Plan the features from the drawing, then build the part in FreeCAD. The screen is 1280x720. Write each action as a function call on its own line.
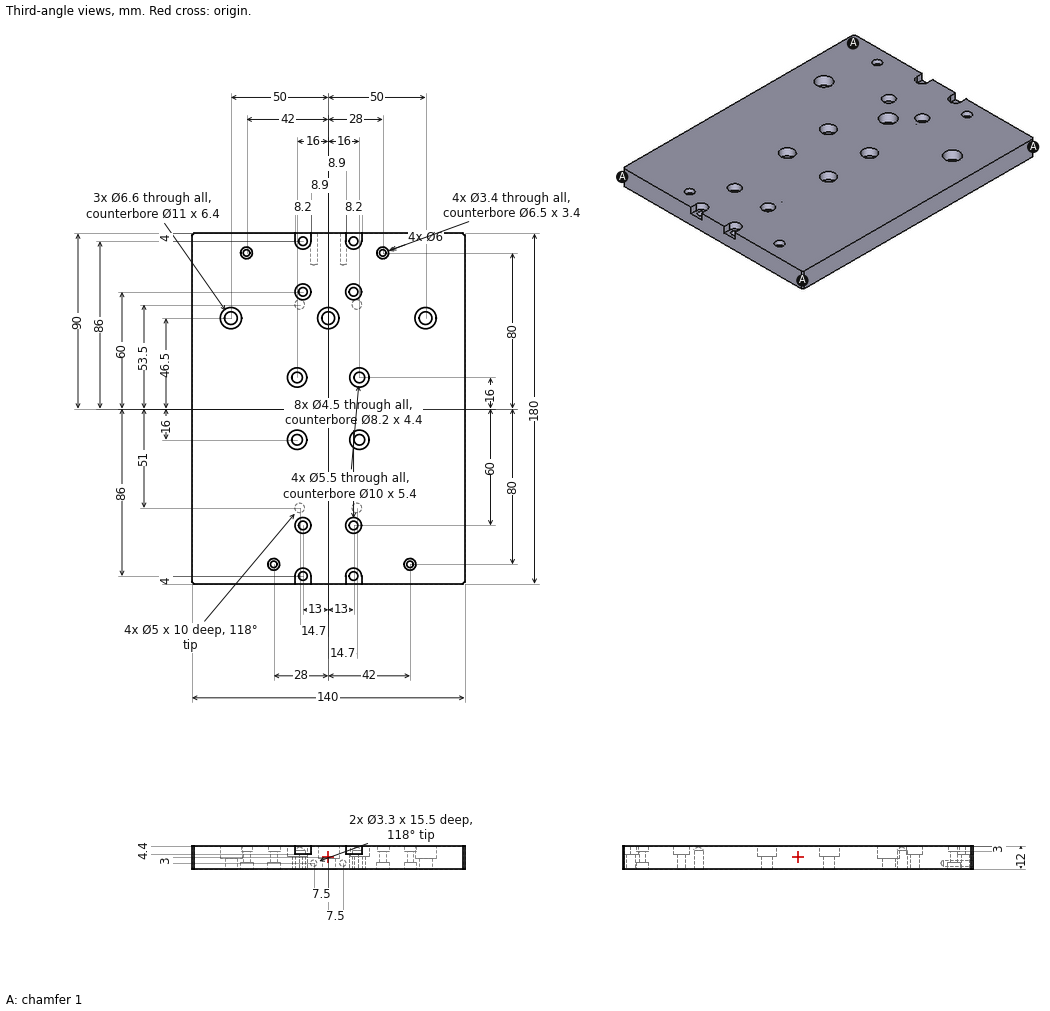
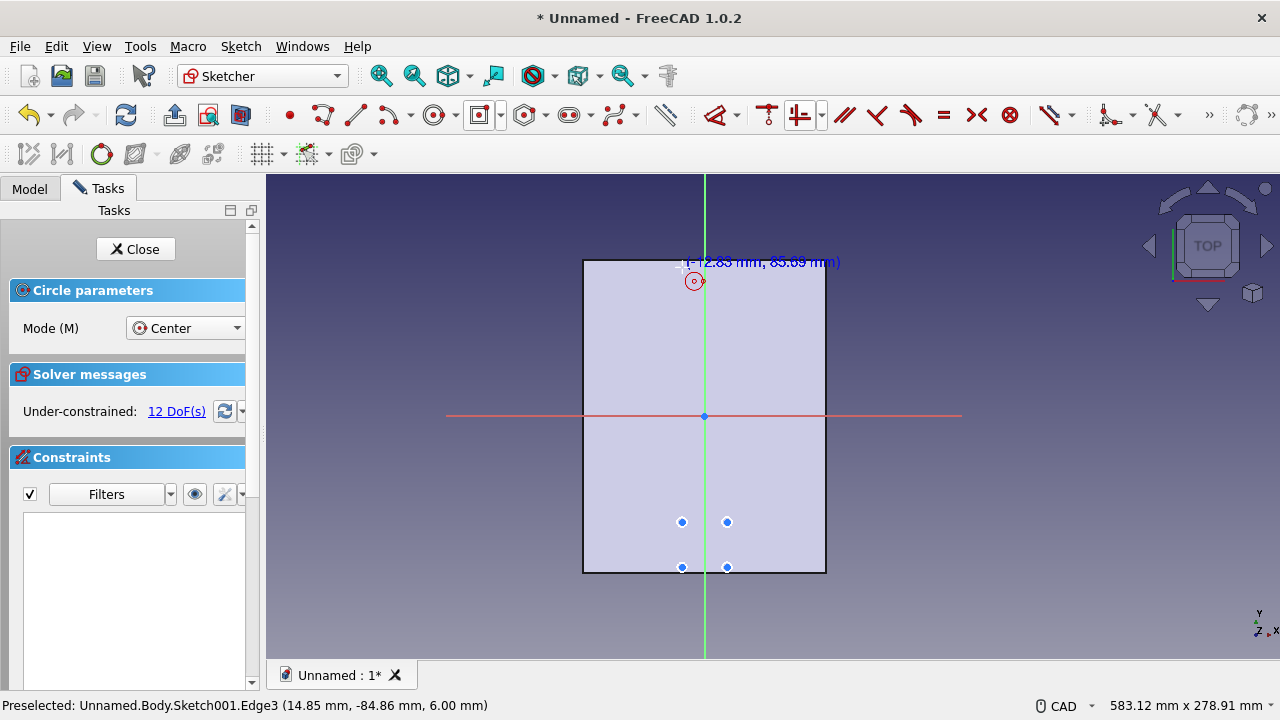
click(682, 267)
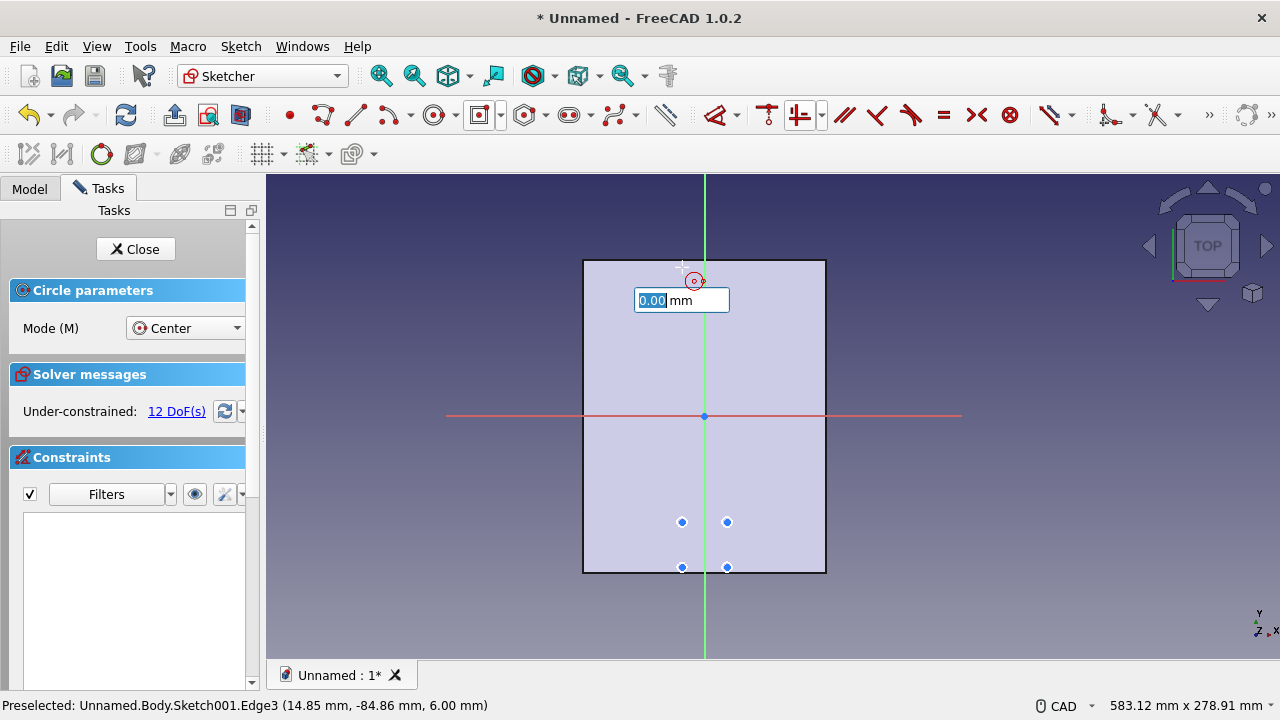
scroll(685, 264, up, 8)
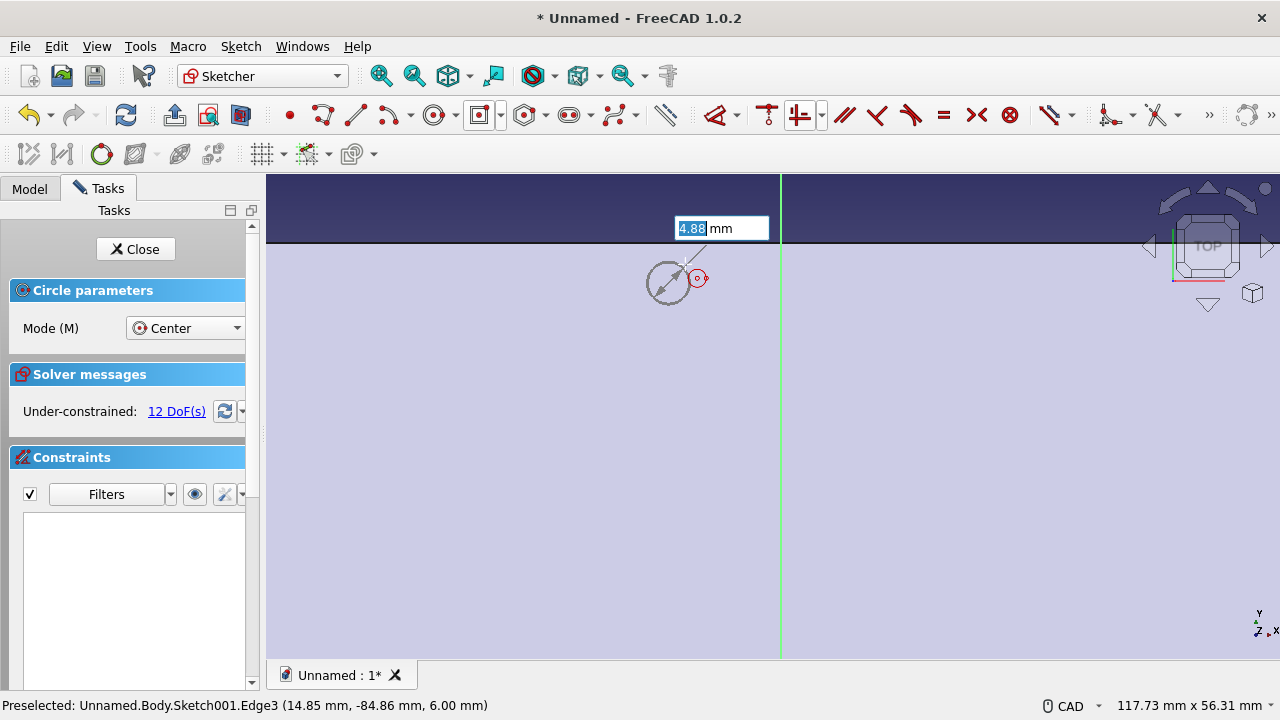
click(682, 263)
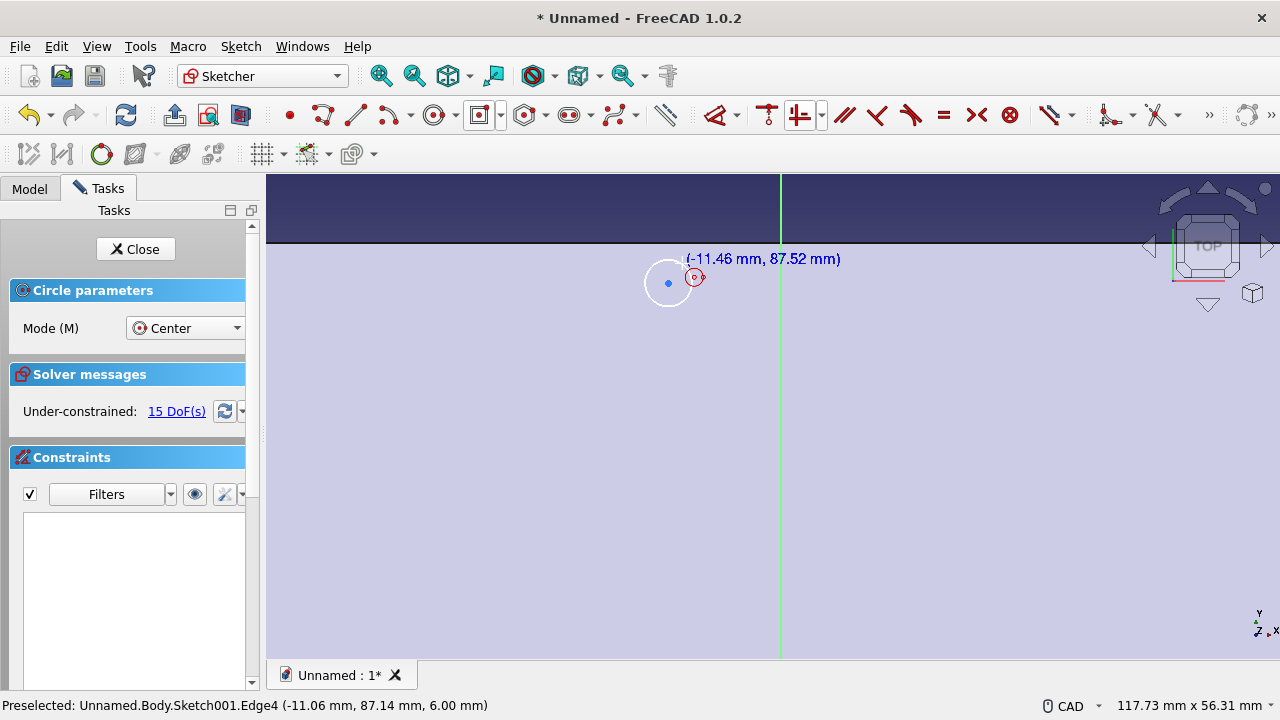
scroll(685, 264, down, 8)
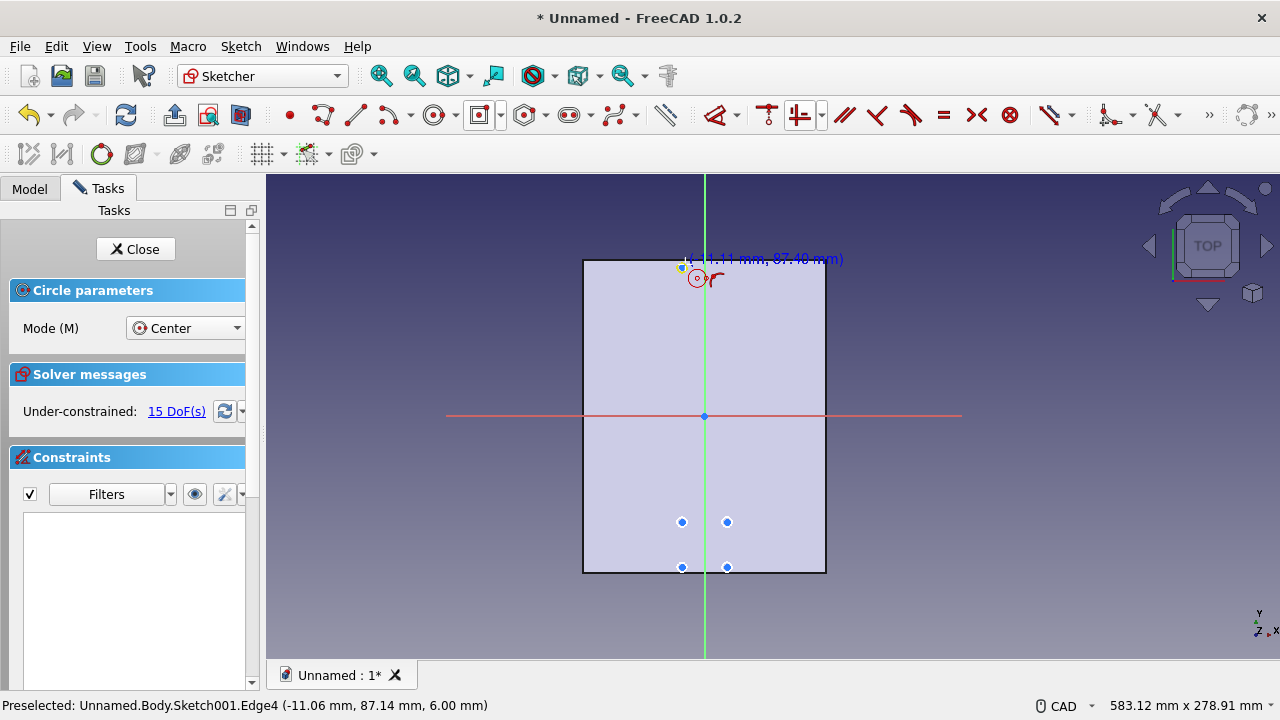
click(727, 267)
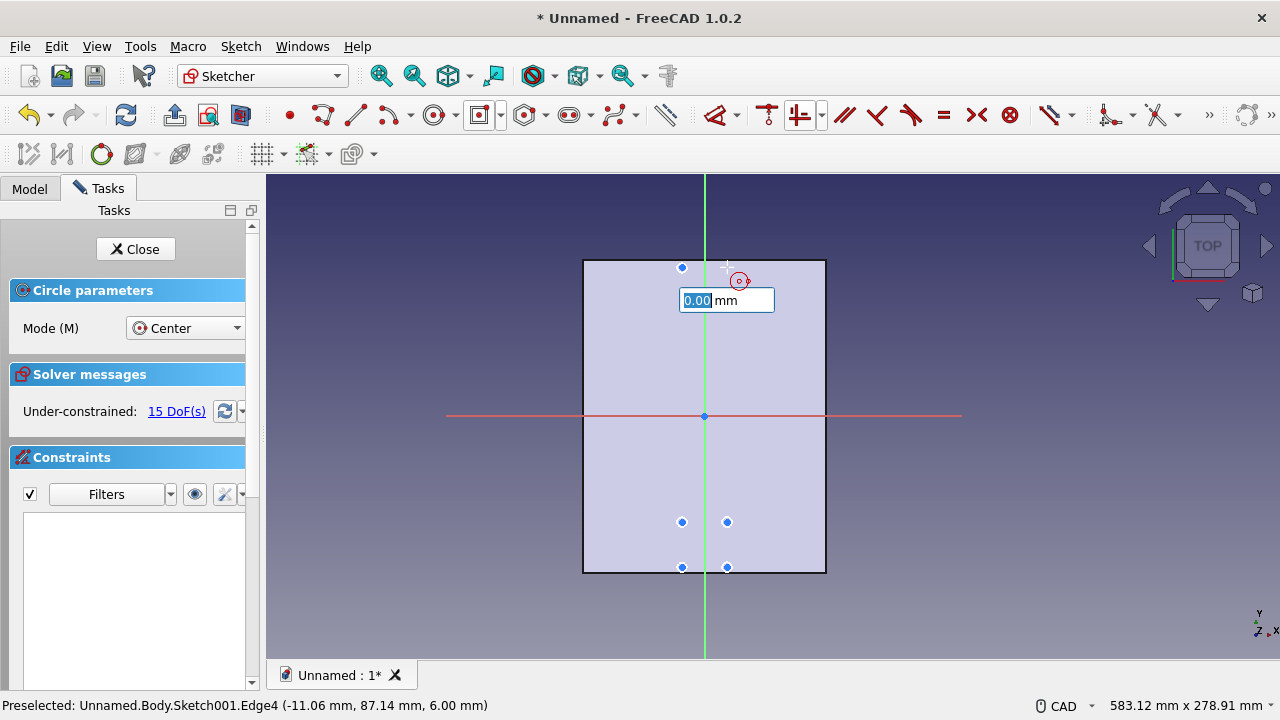
scroll(730, 264, up, 8)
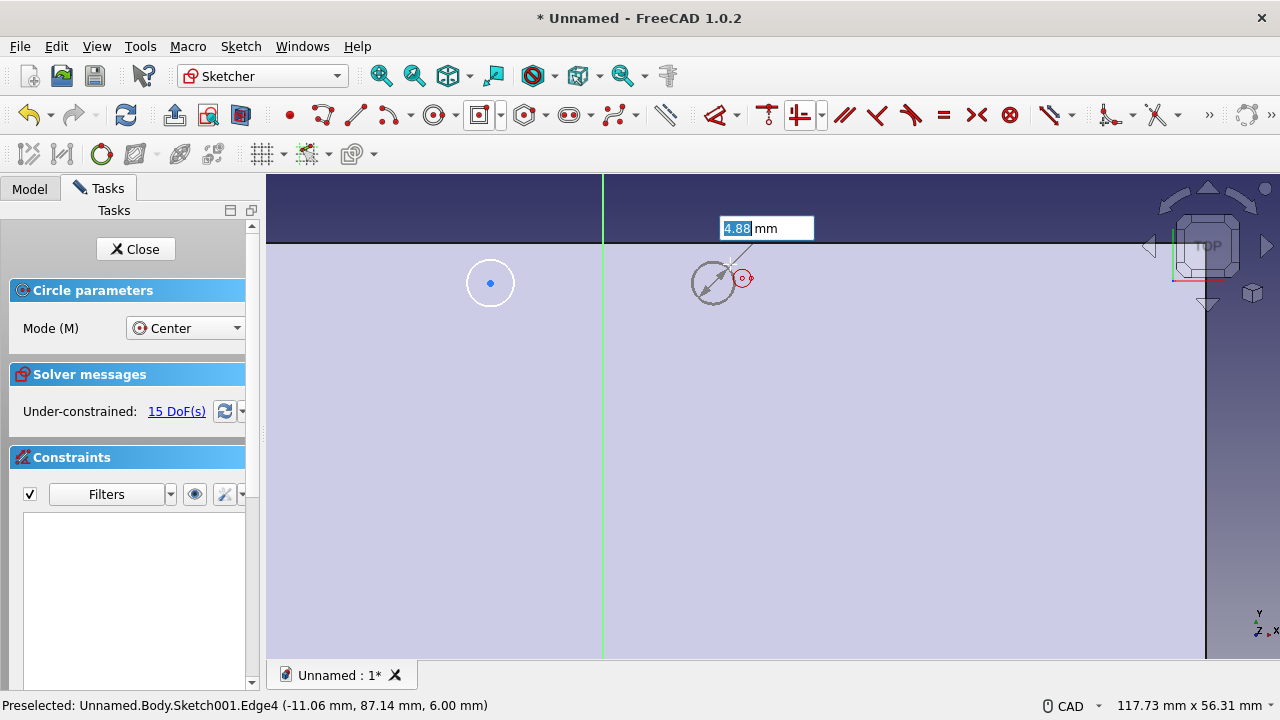
click(728, 263)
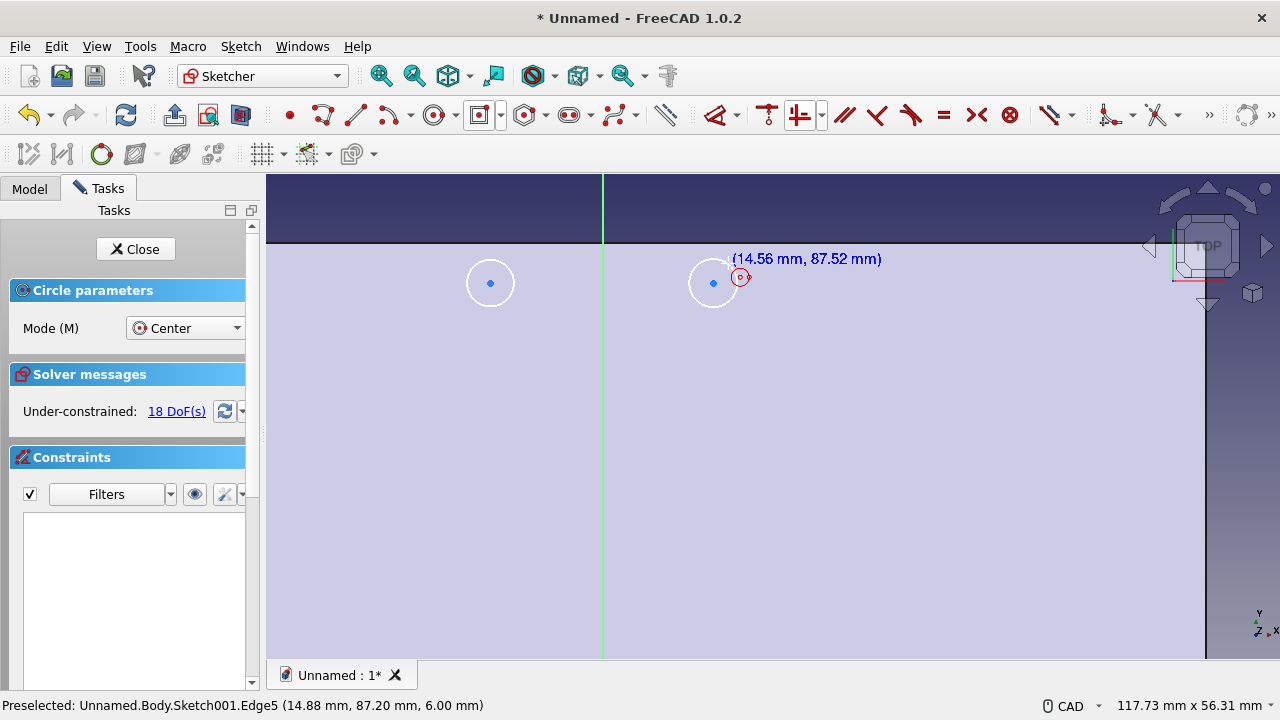
scroll(730, 264, down, 8)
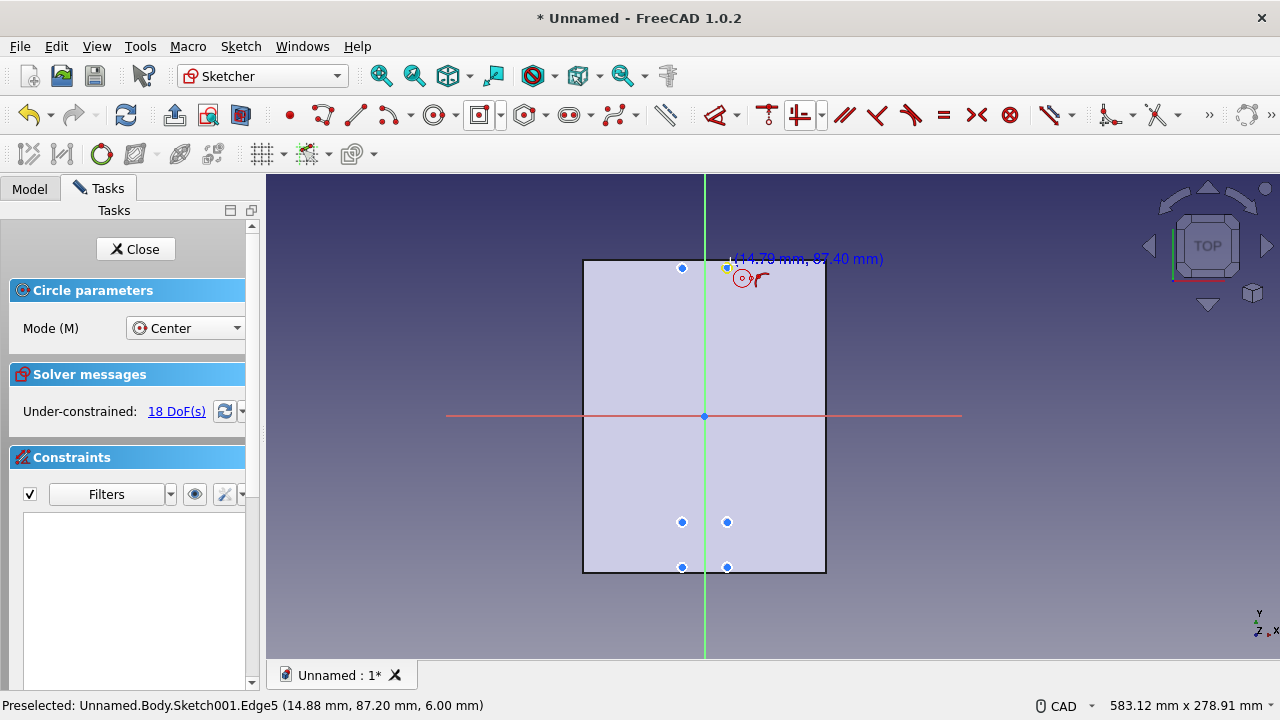
click(682, 312)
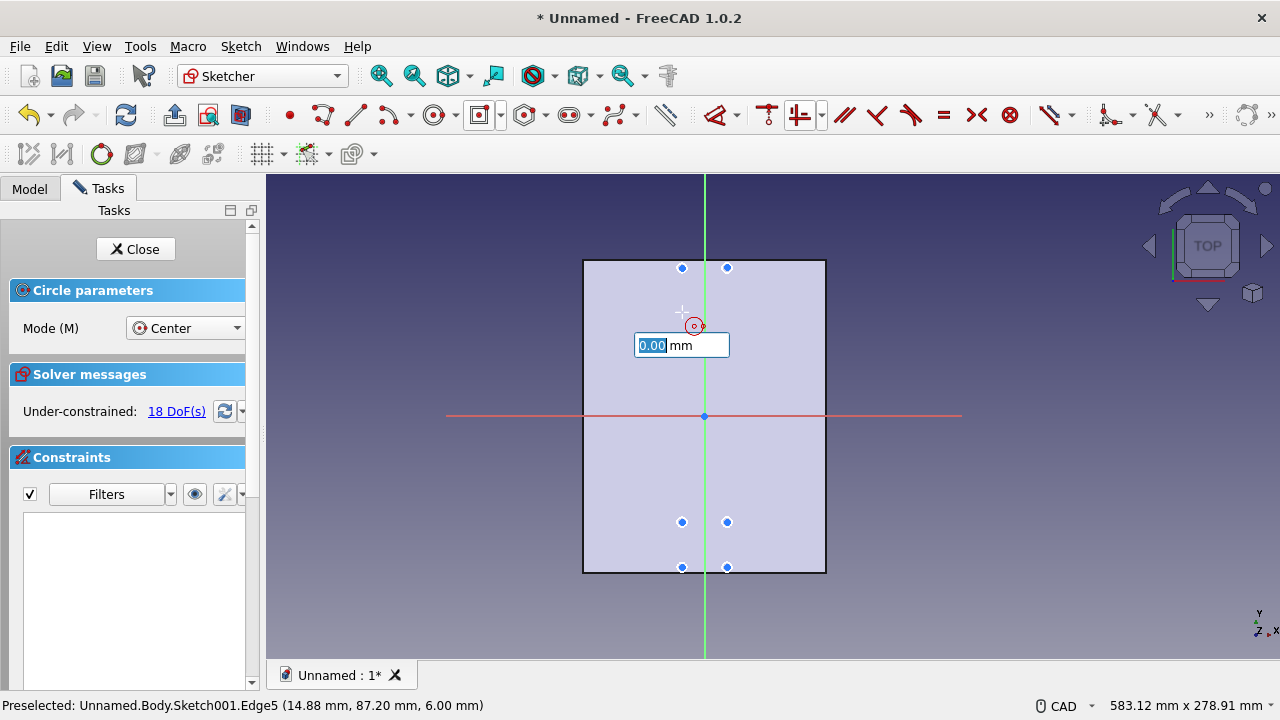
scroll(685, 309, up, 8)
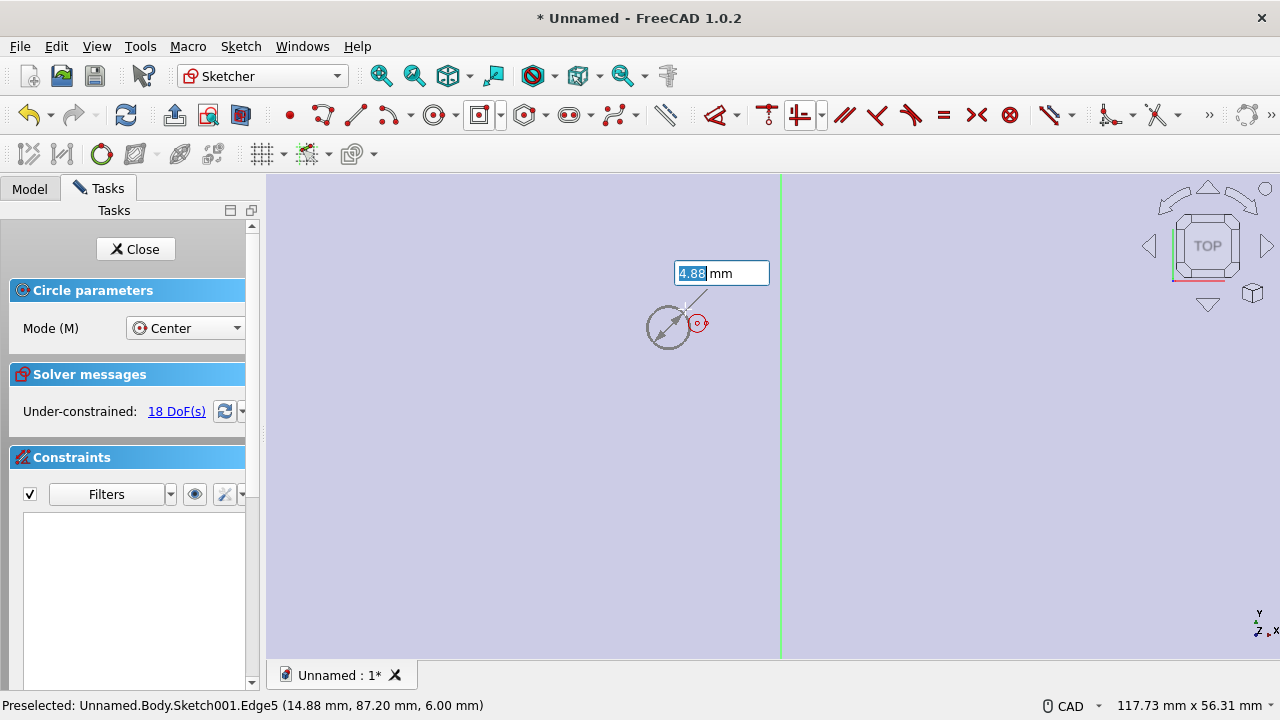
click(682, 309)